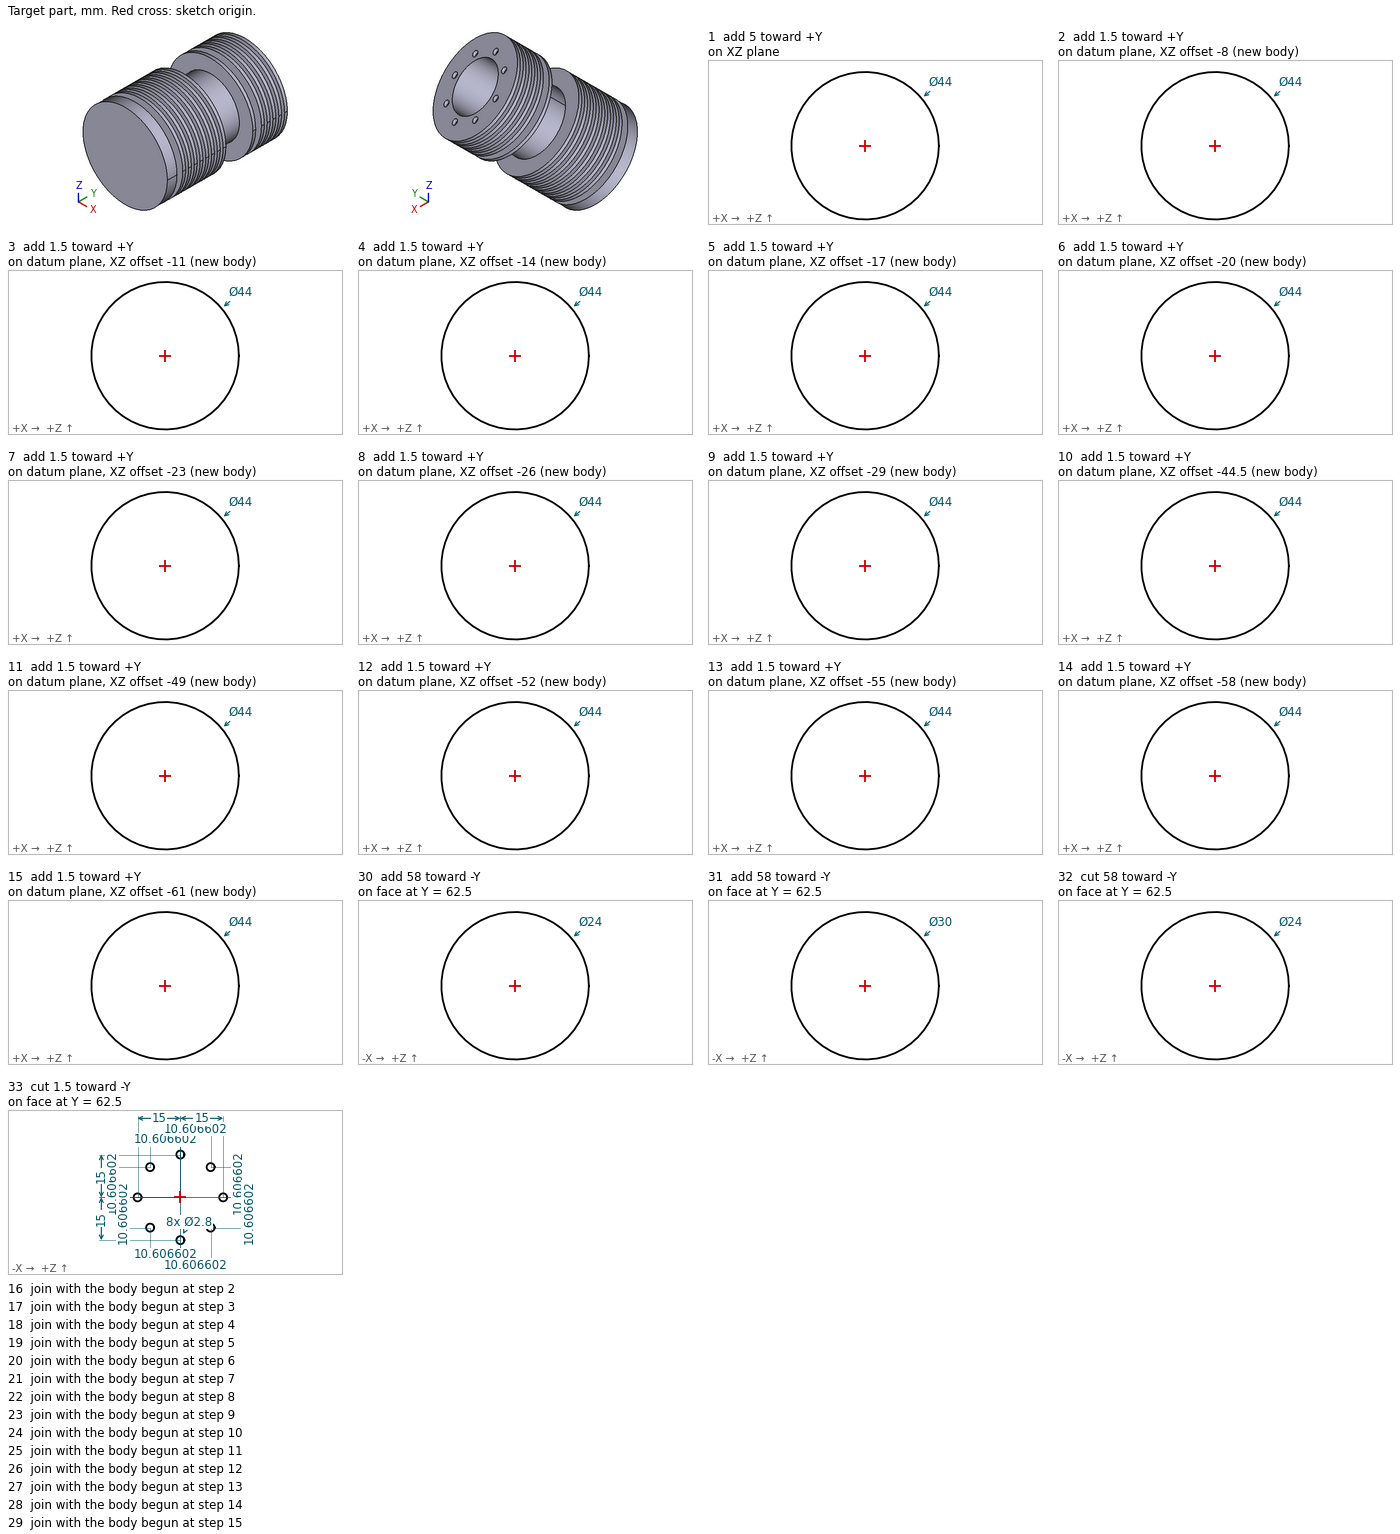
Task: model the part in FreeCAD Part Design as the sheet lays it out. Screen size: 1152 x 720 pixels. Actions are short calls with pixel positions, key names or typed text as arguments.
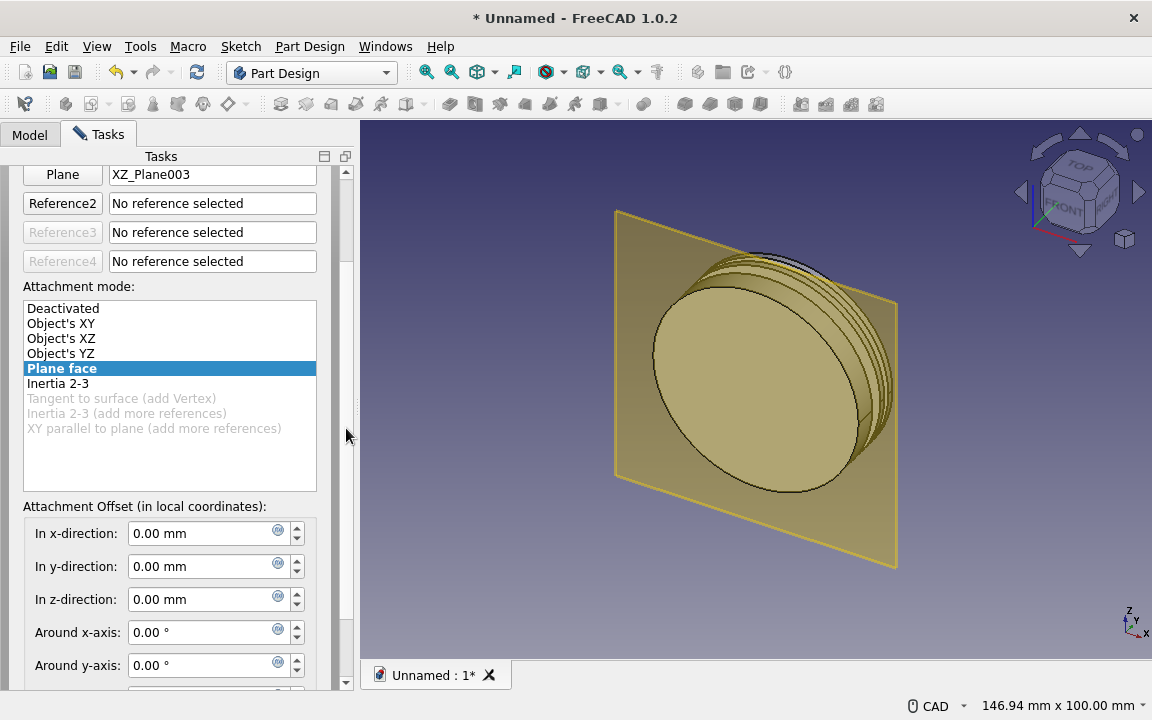
triple_click(210, 600)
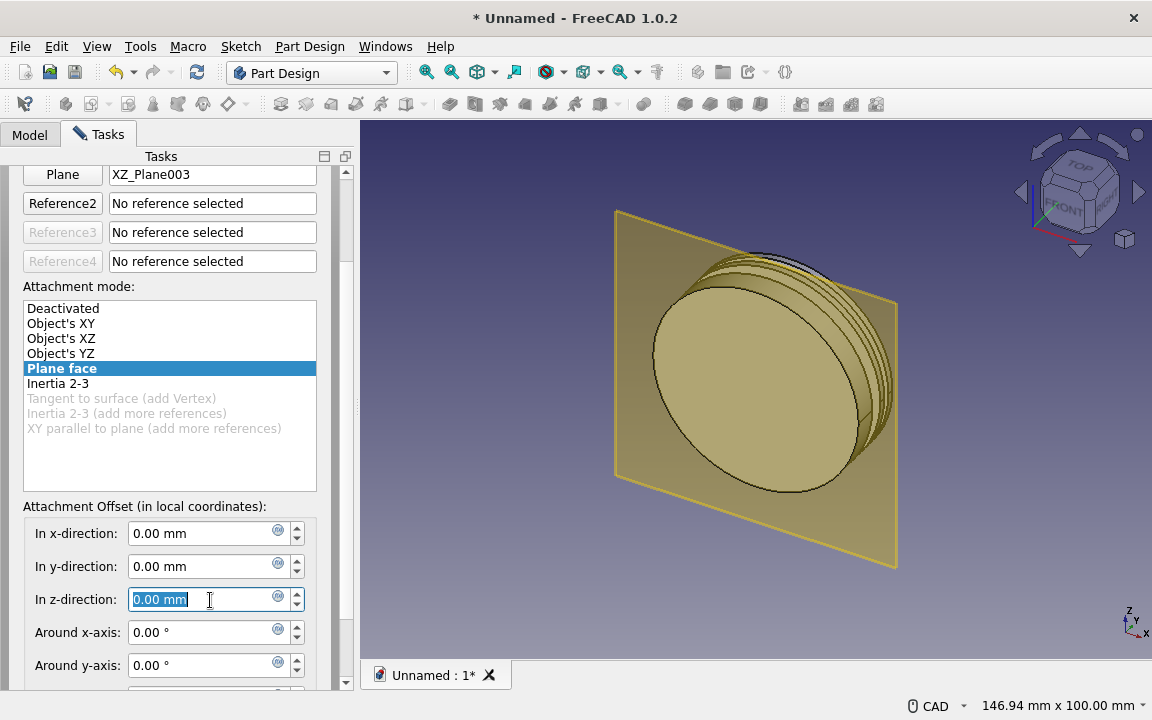
text(-14)
key(Tab)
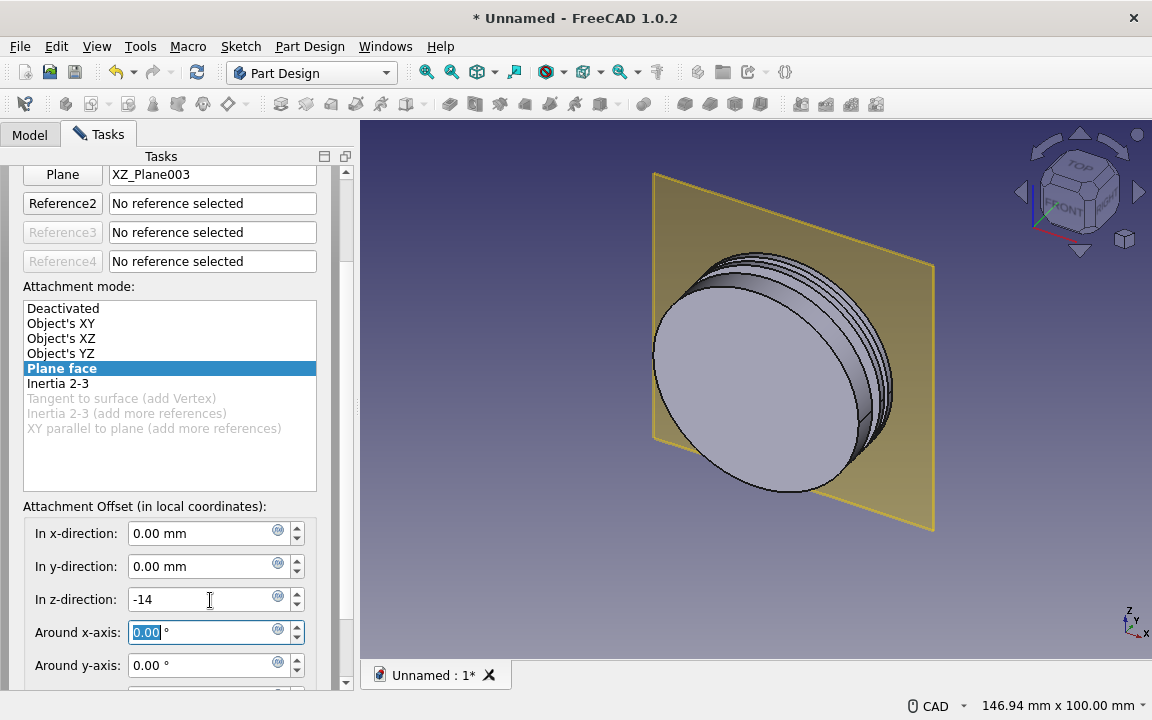
scroll(346, 428, up, 3)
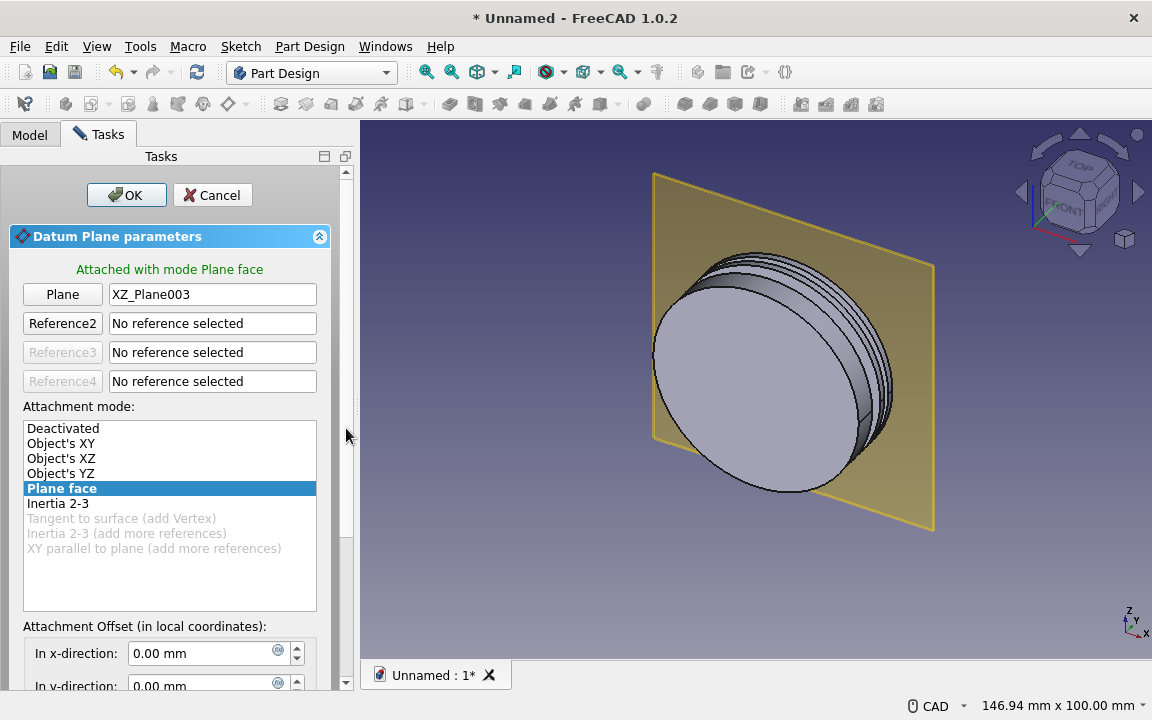
click(127, 195)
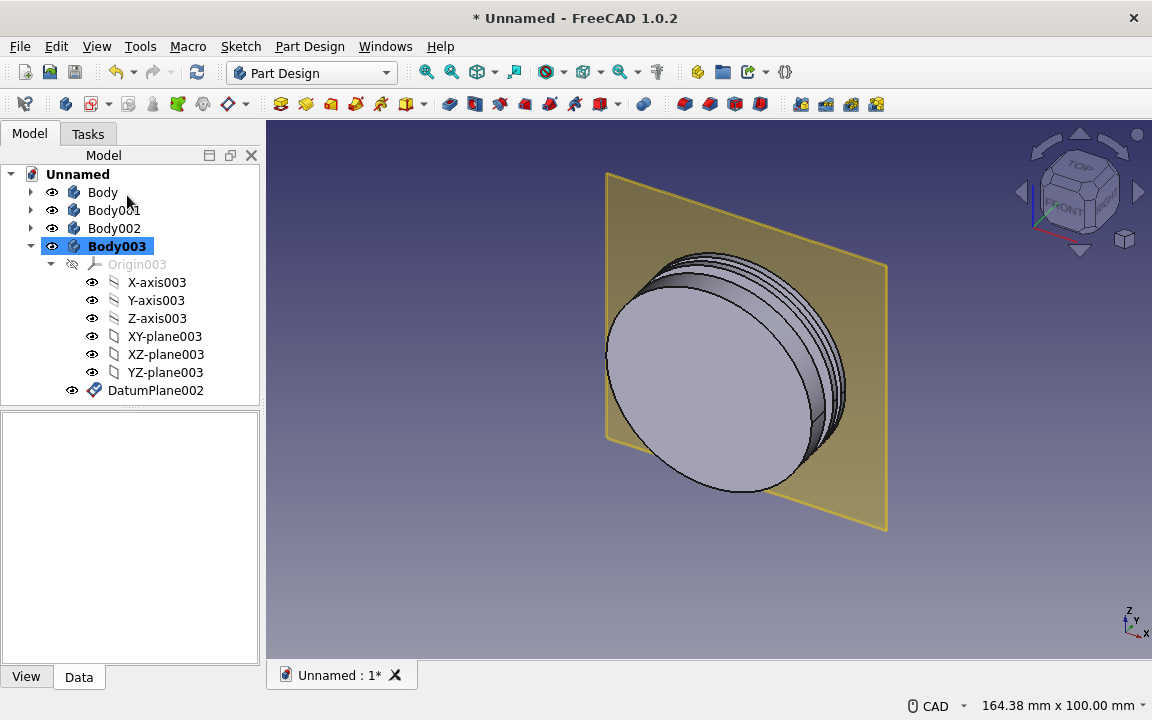
click(117, 390)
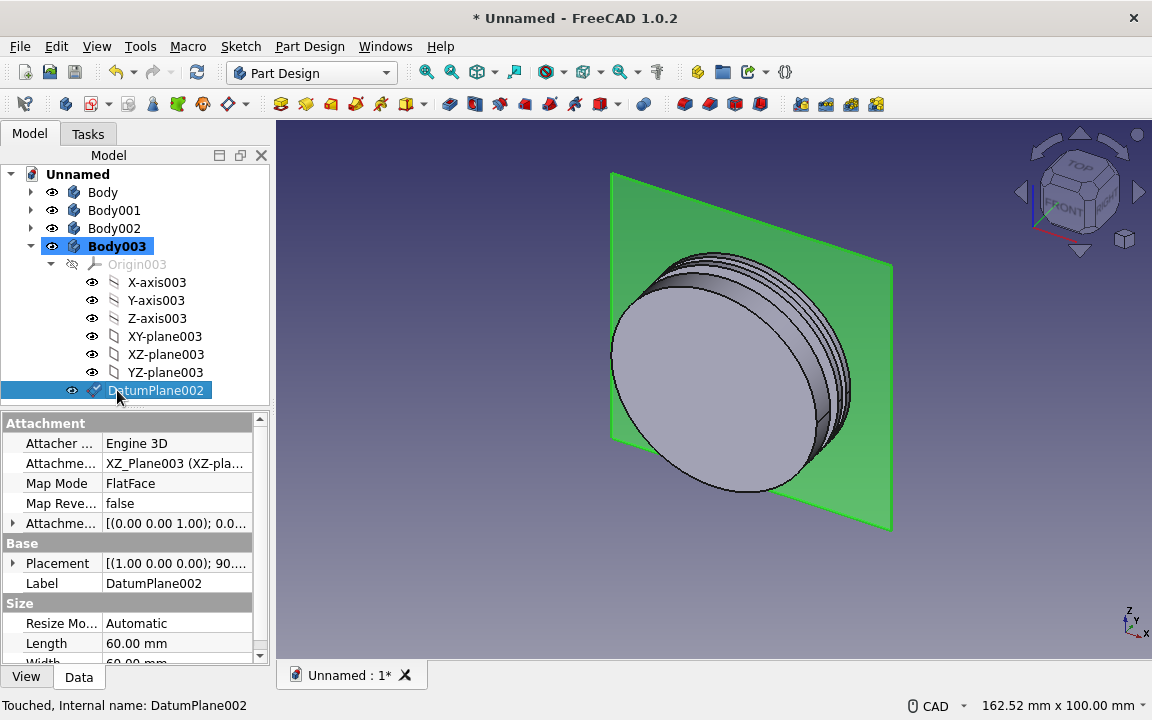
click(90, 104)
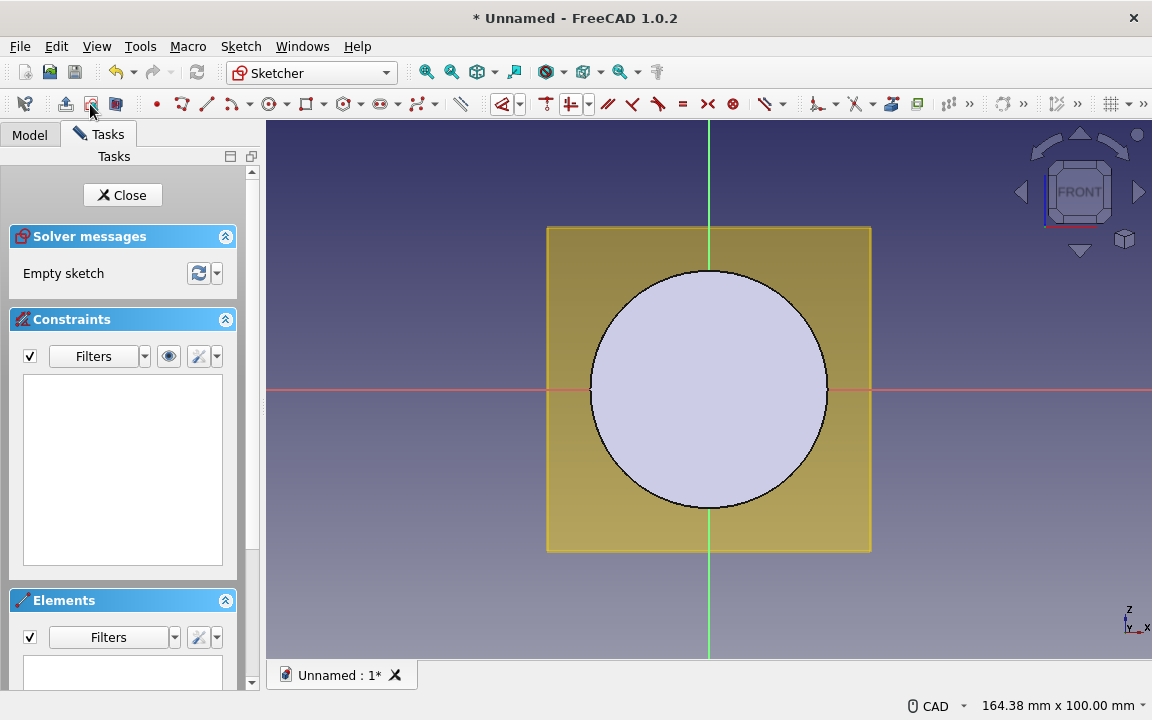
scroll(848, 390, up, 2)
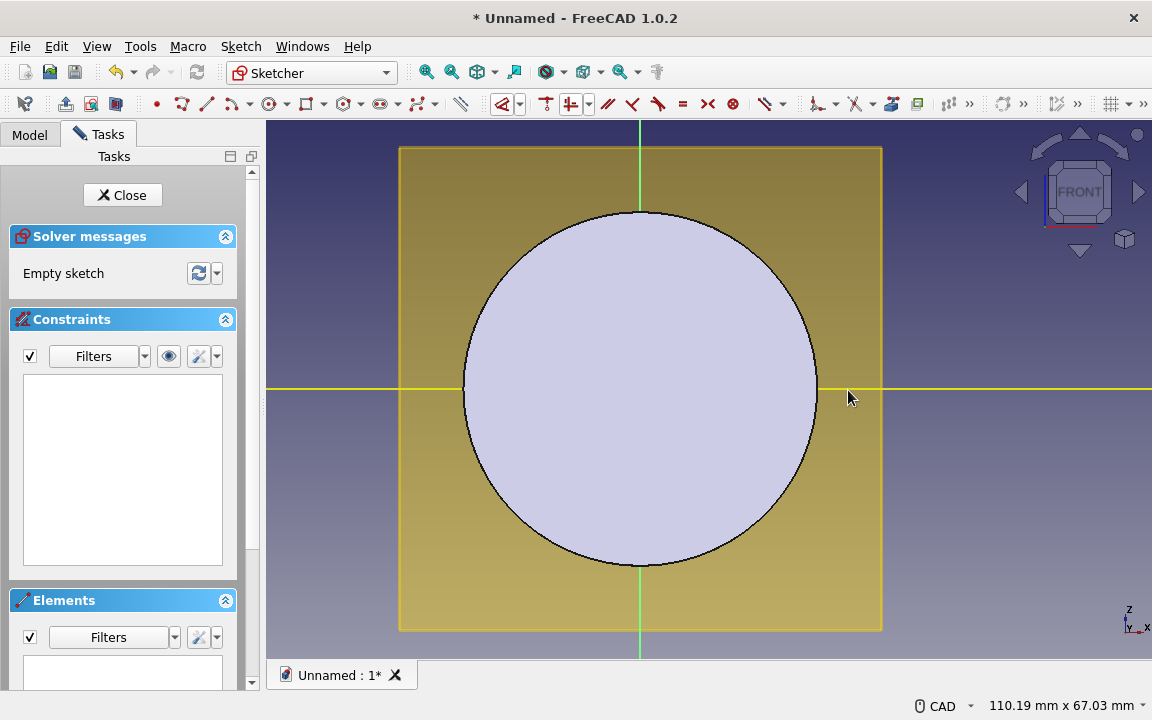
click(268, 104)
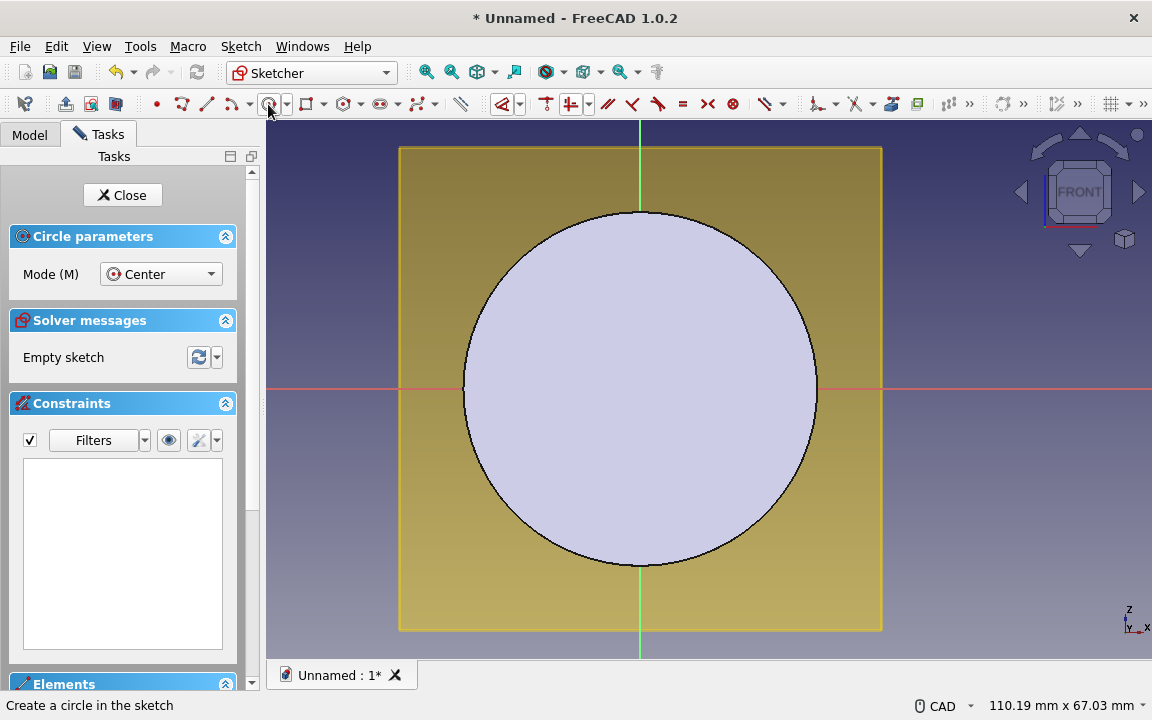
click(640, 389)
click(765, 264)
key(Escape)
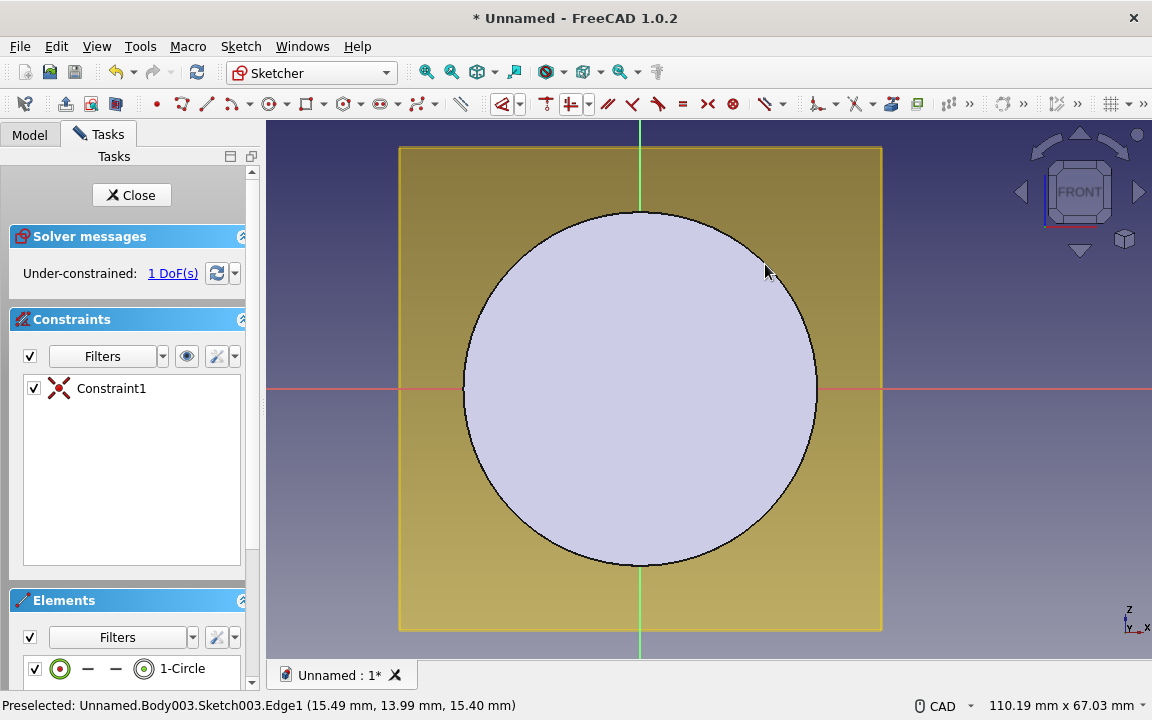
click(764, 264)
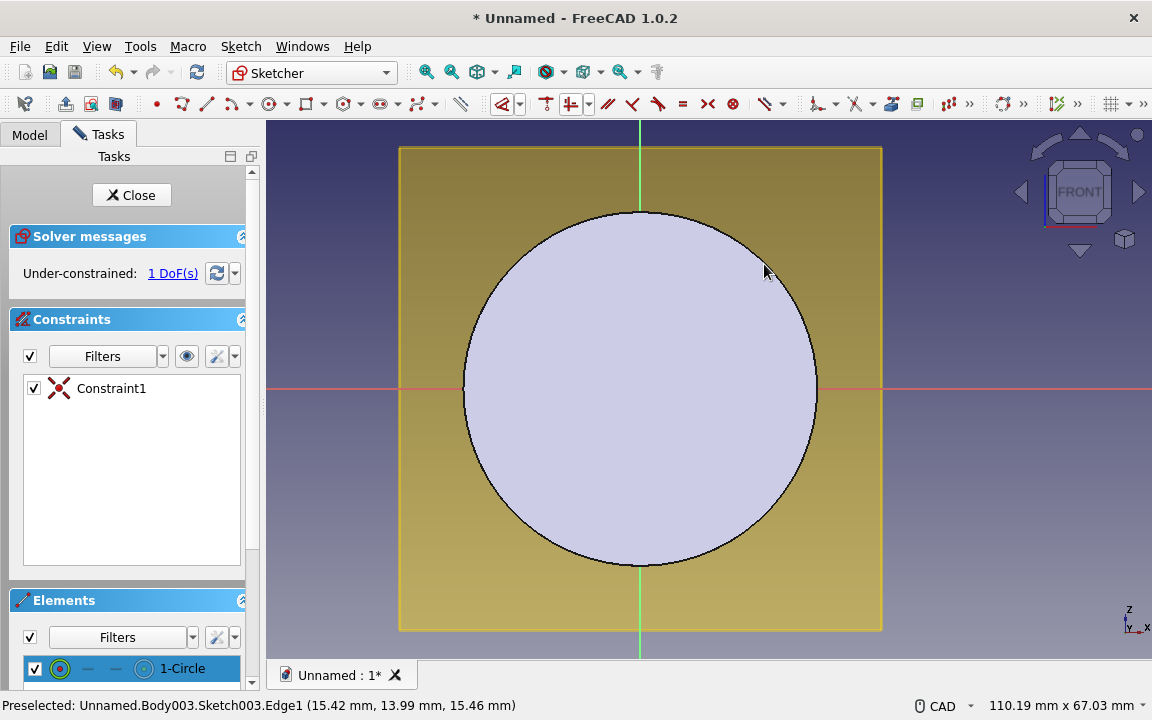
key(k)
key(o)